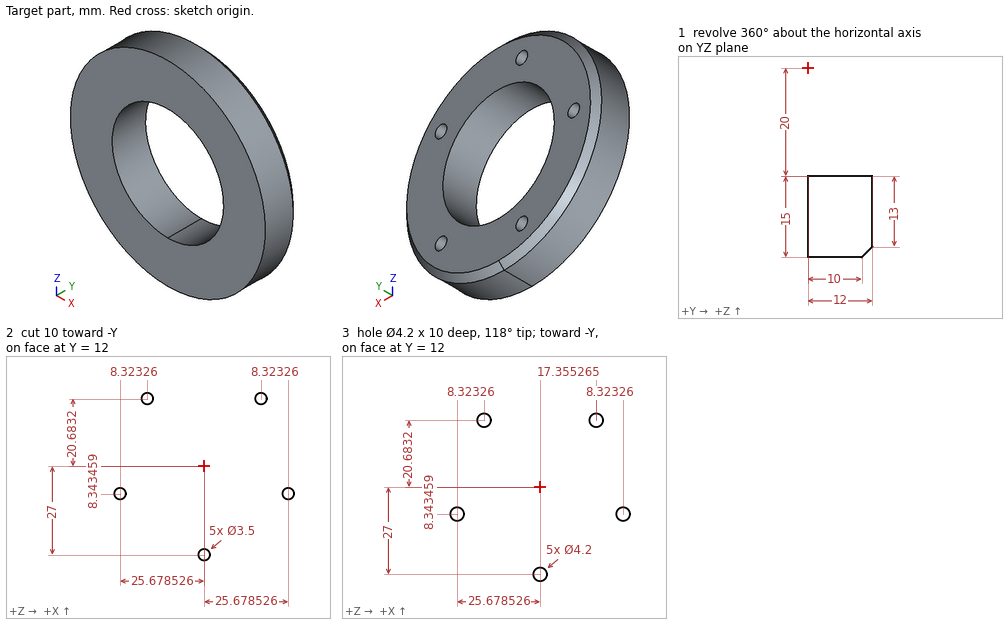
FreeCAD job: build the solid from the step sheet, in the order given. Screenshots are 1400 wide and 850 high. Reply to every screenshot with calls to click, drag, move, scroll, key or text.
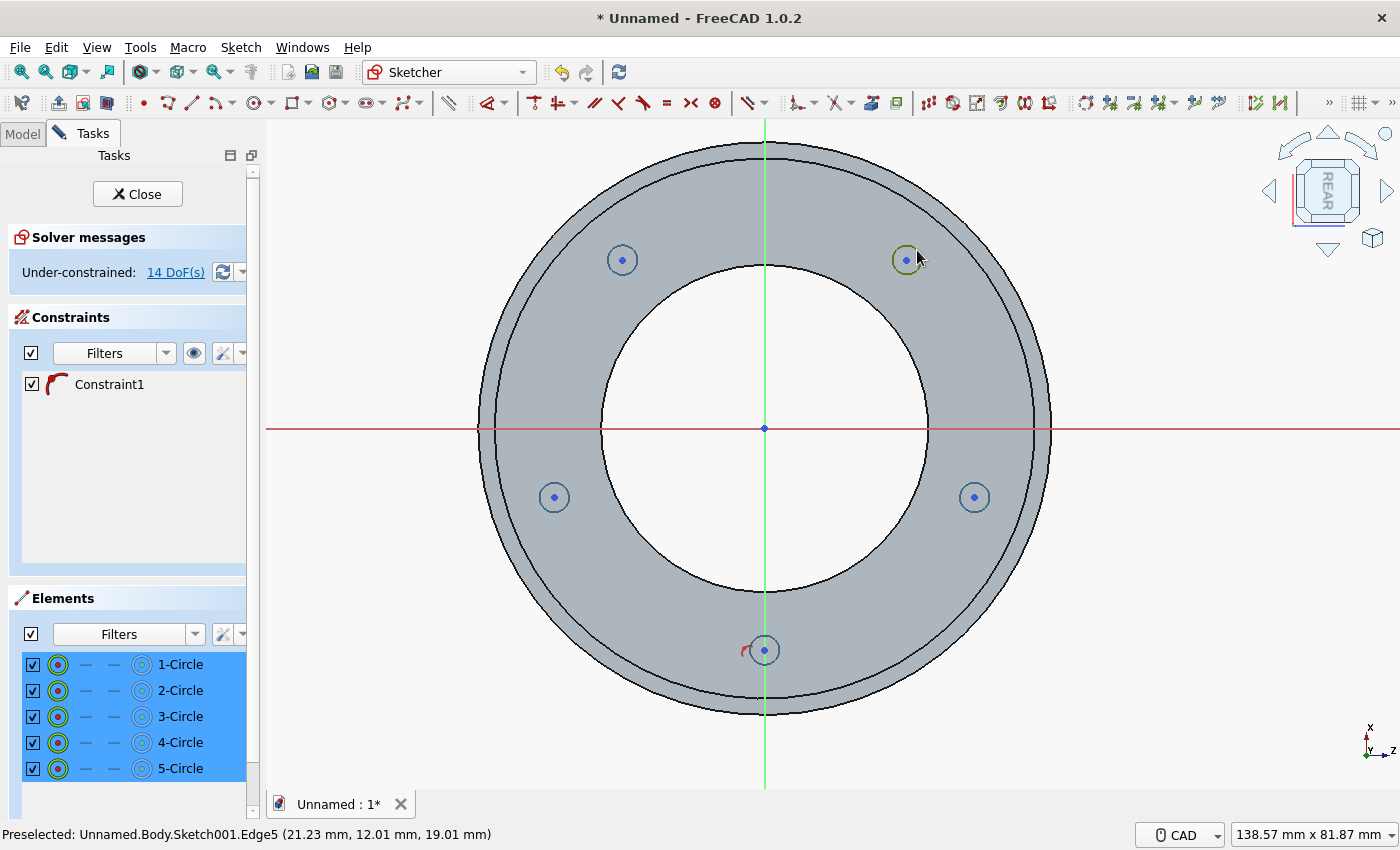
click(668, 104)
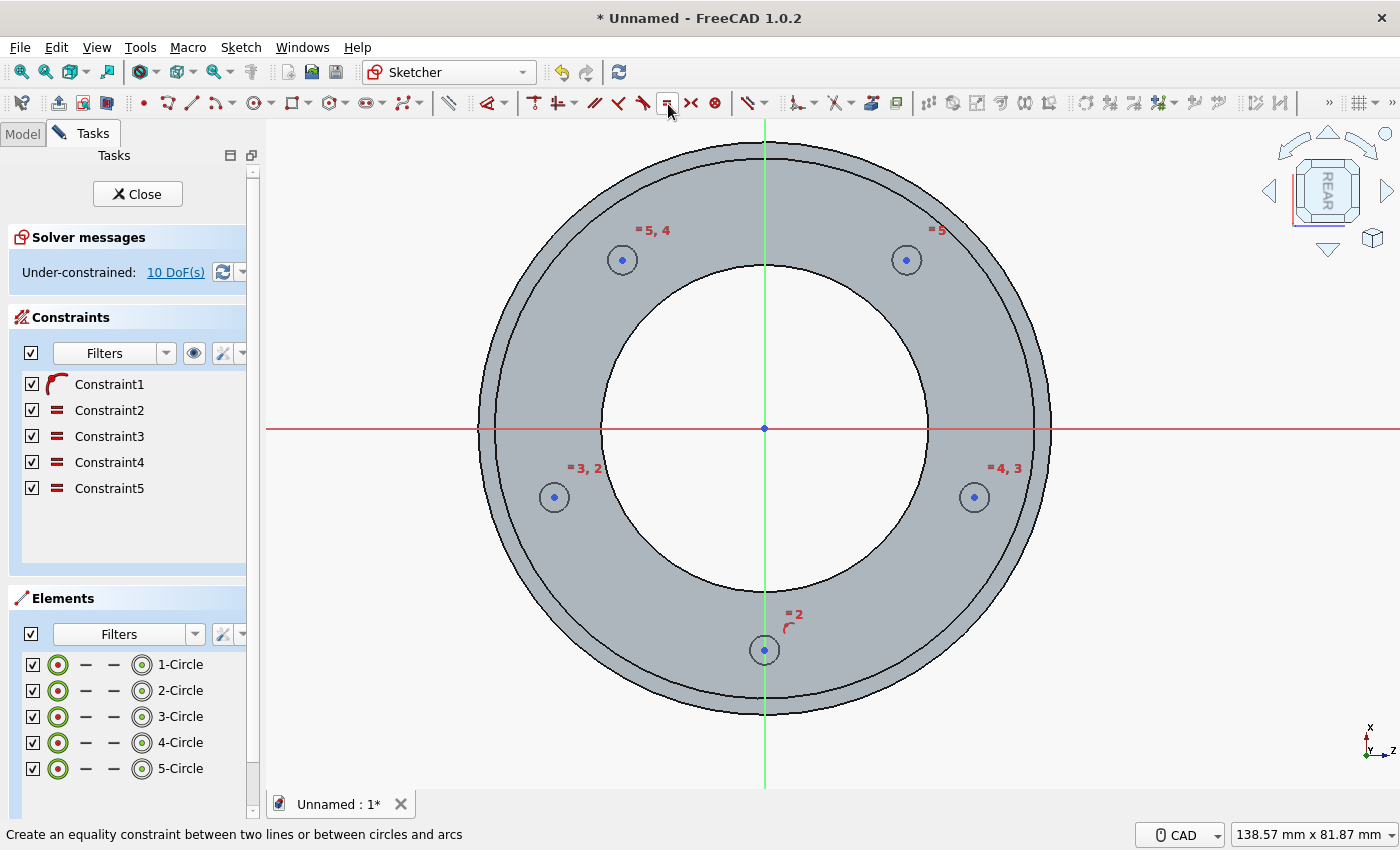
click(554, 498)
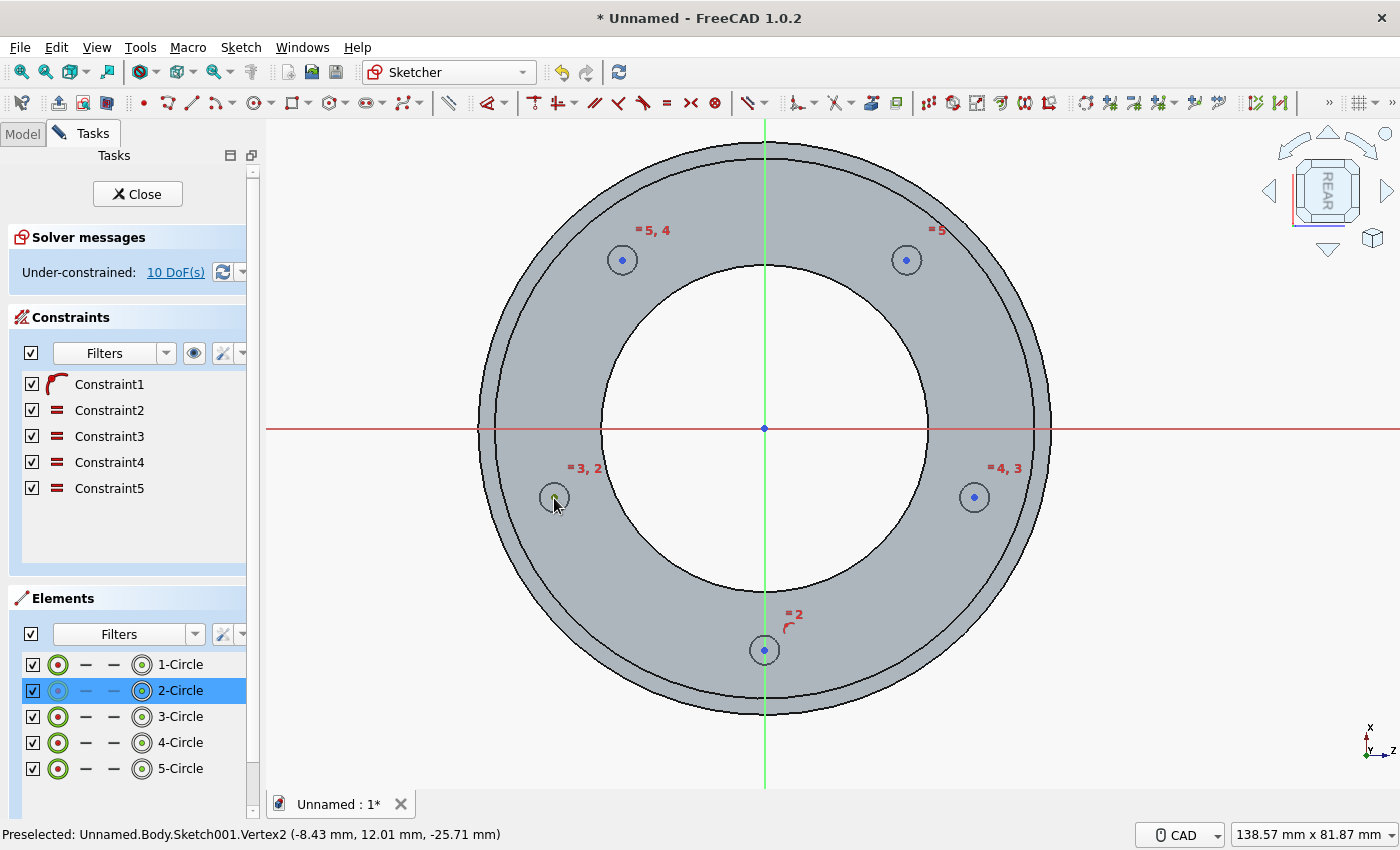
click(975, 498)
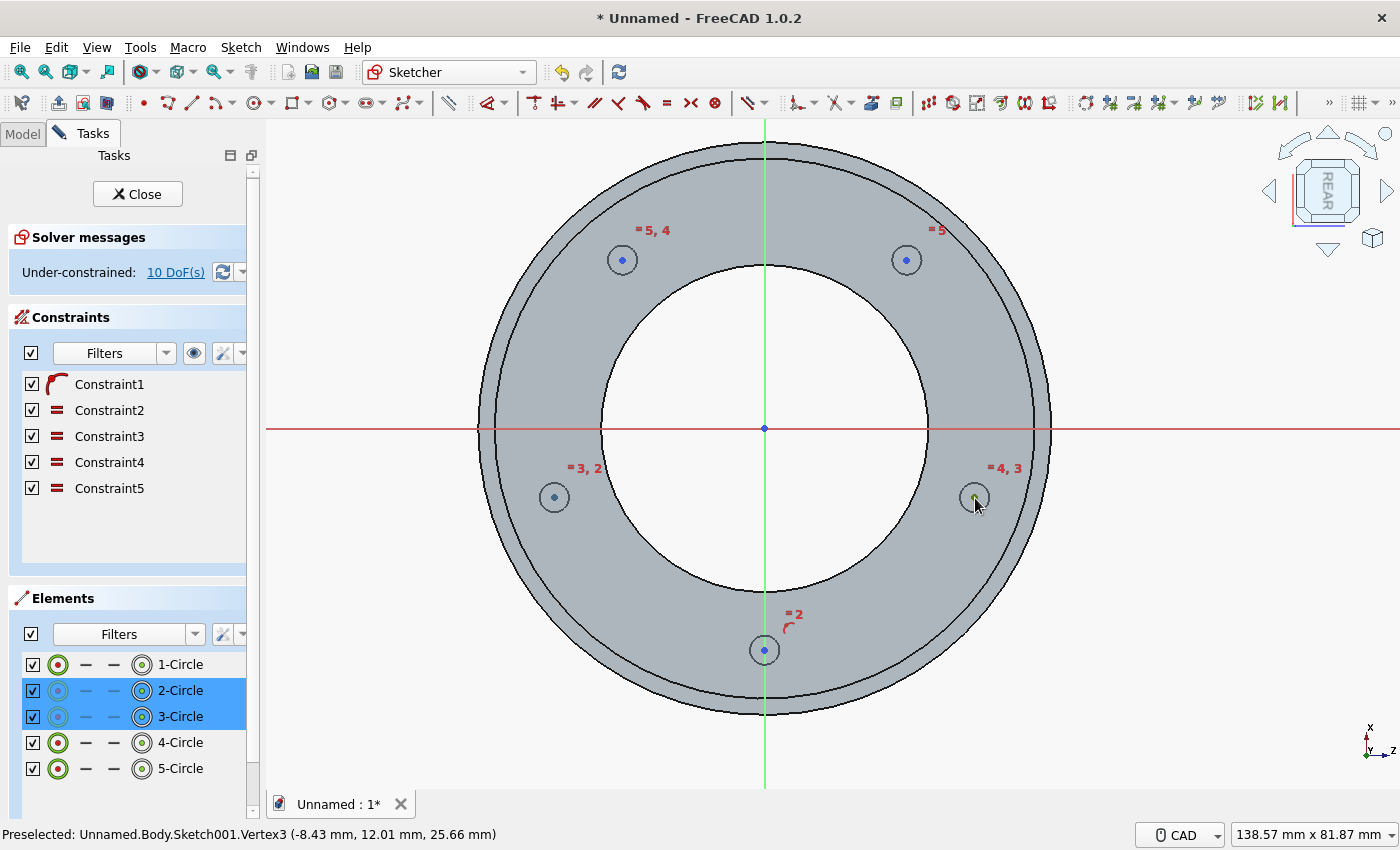
click(576, 104)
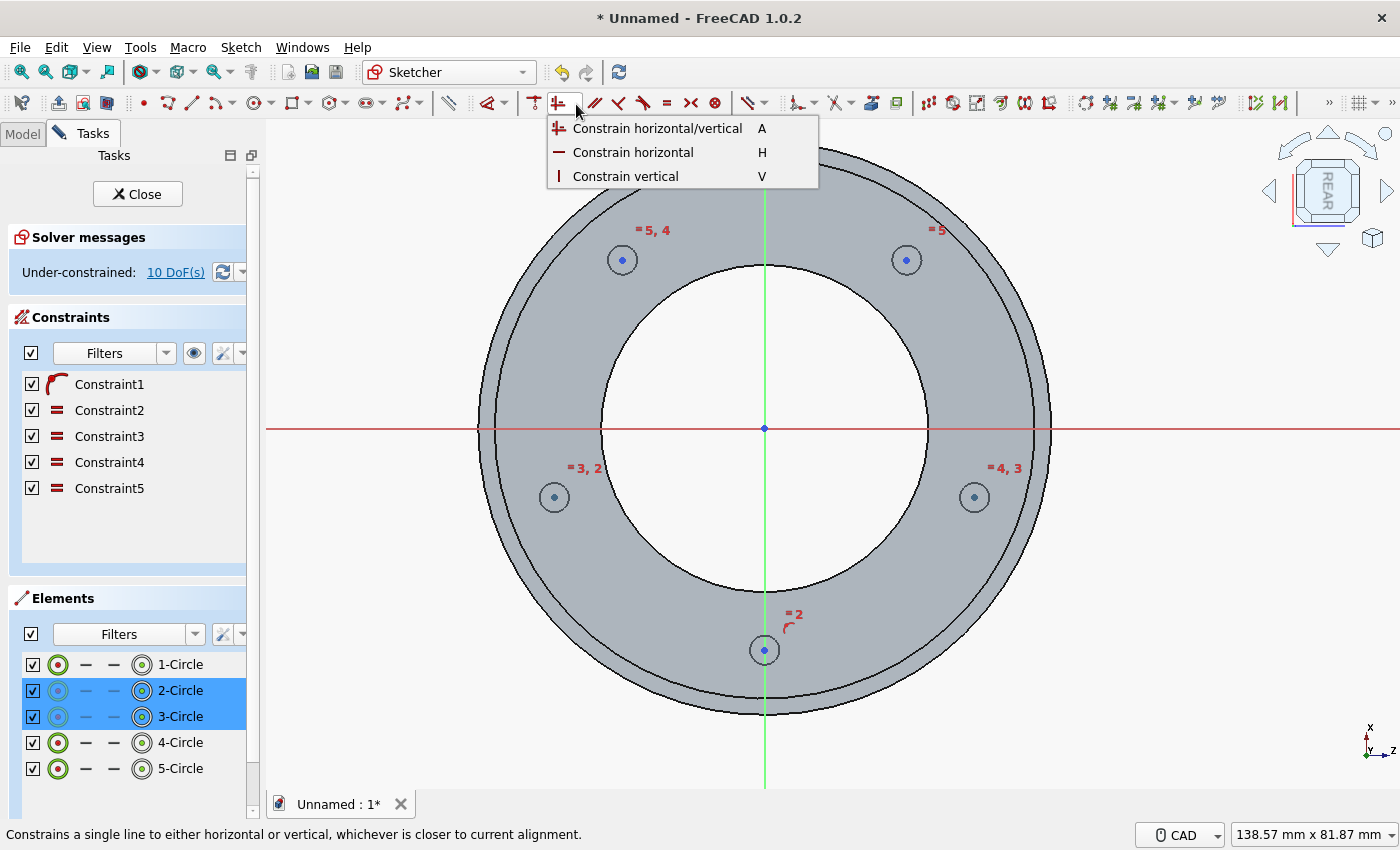
click(683, 152)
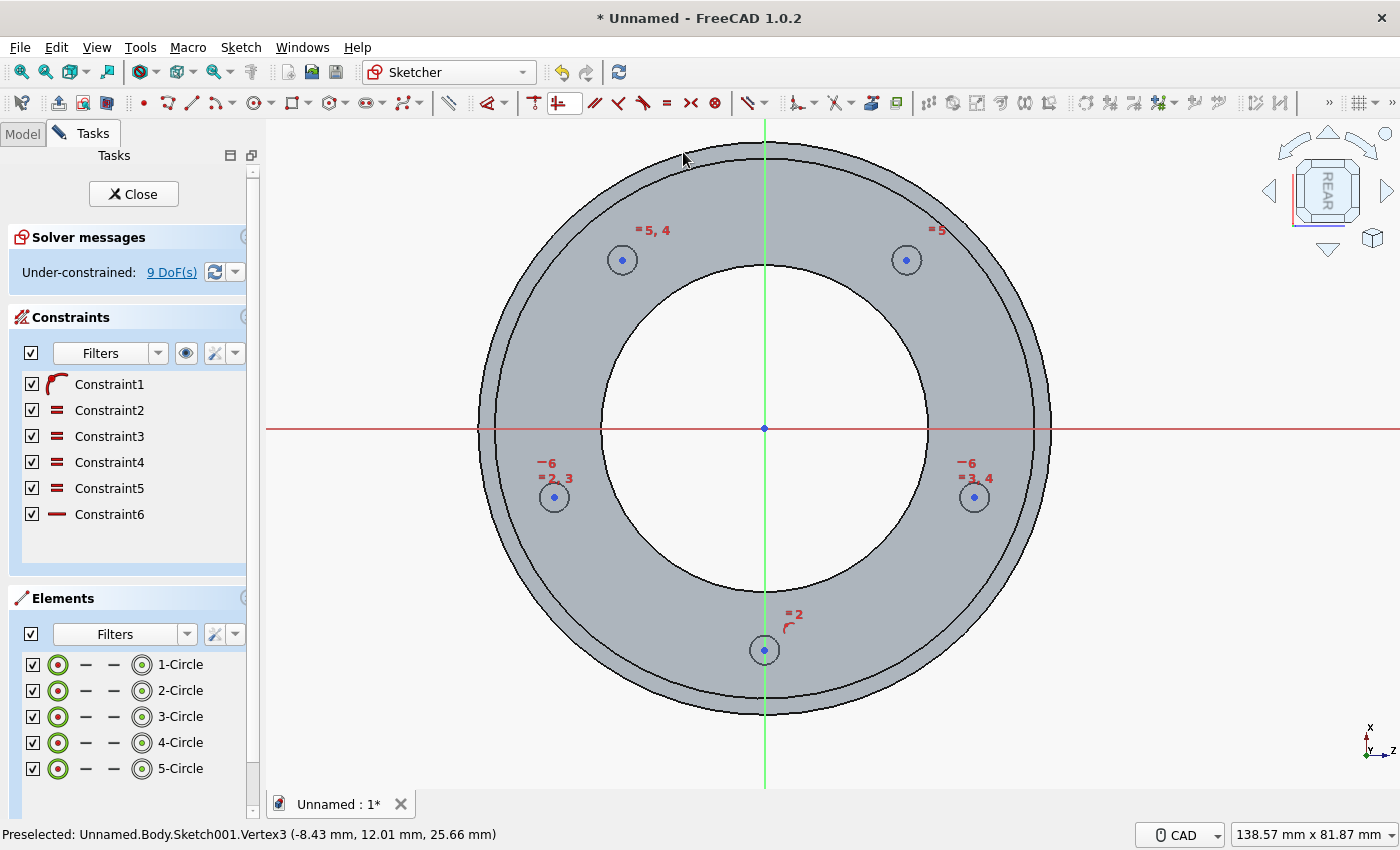
click(623, 260)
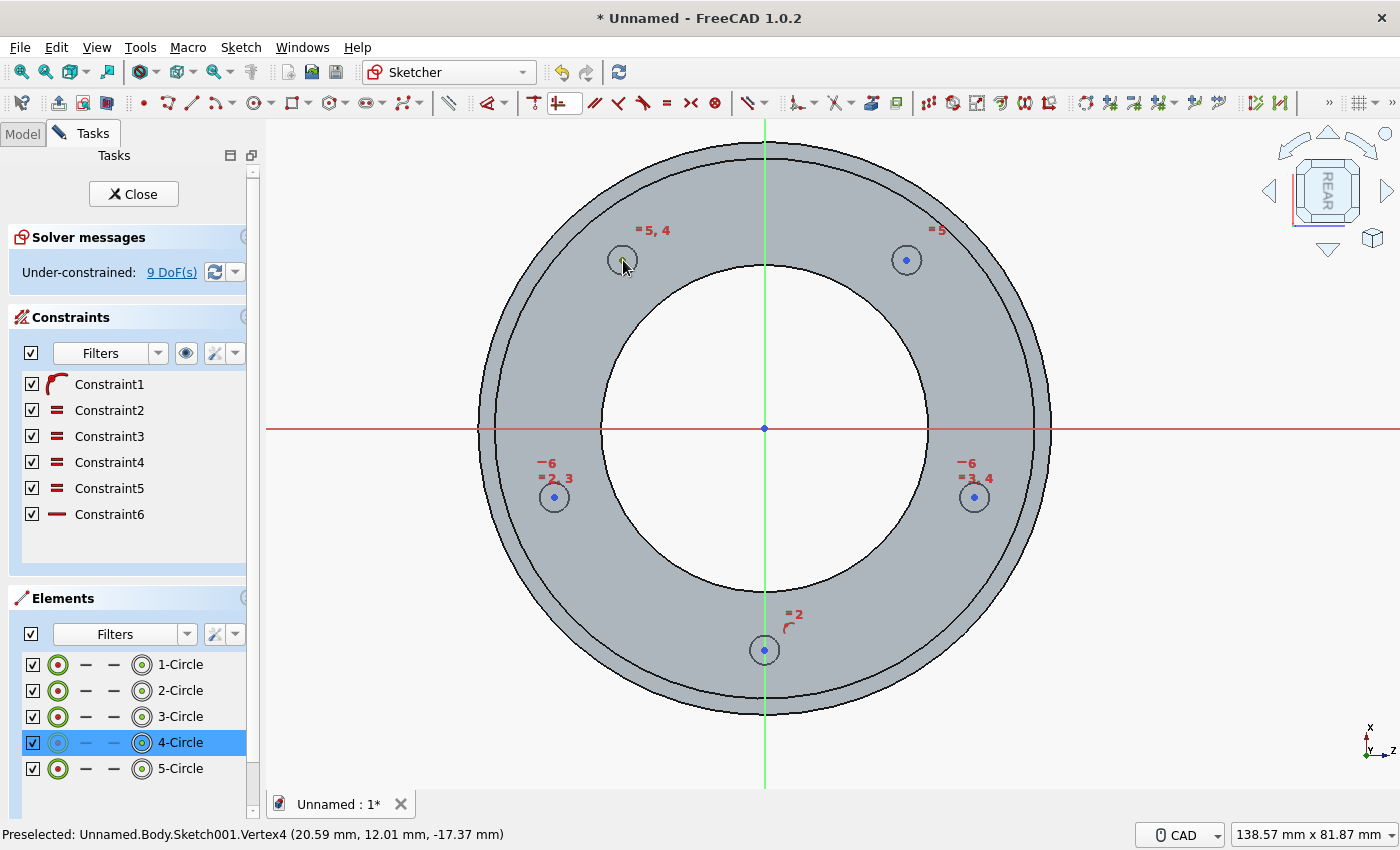
click(907, 260)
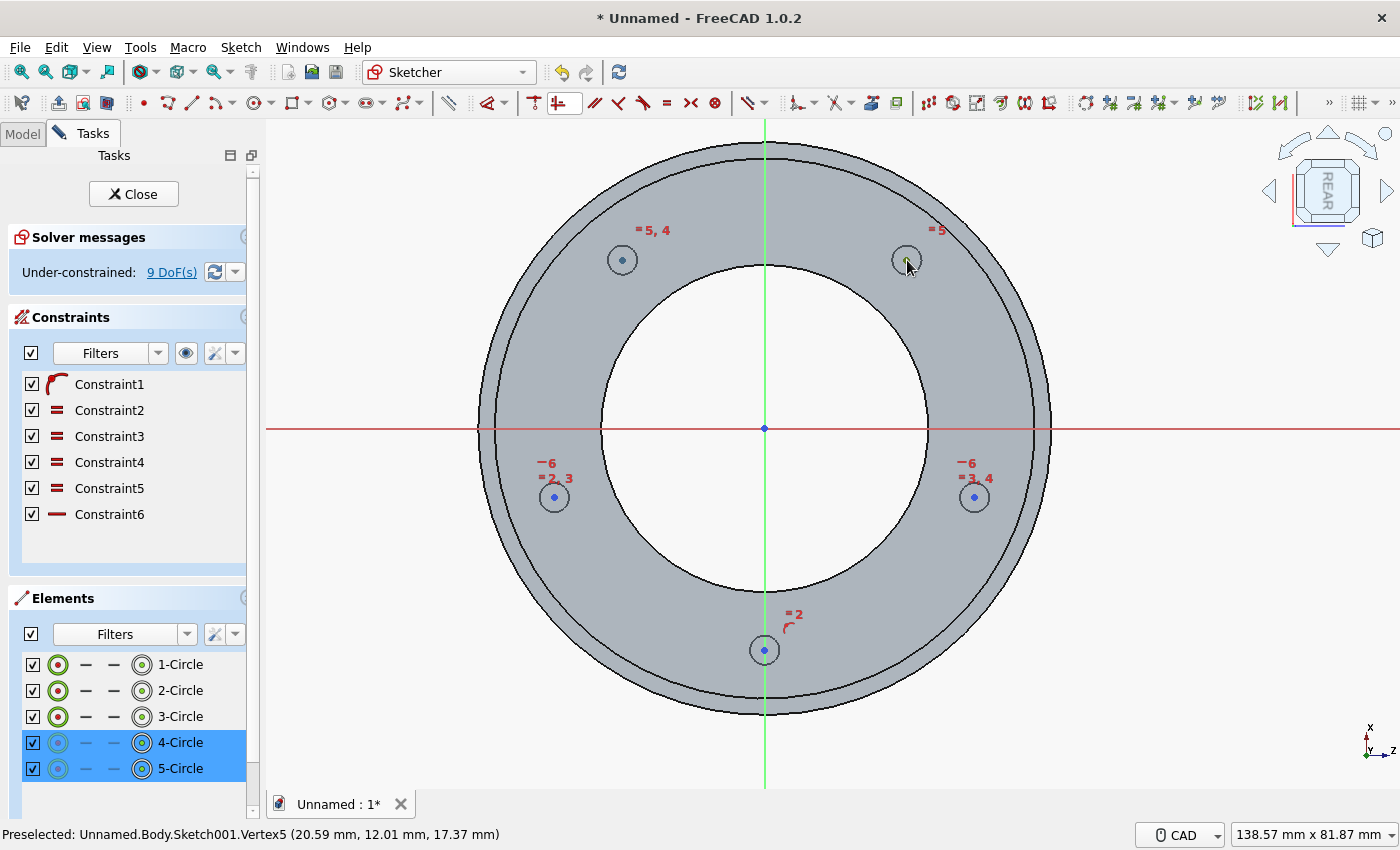
key(h)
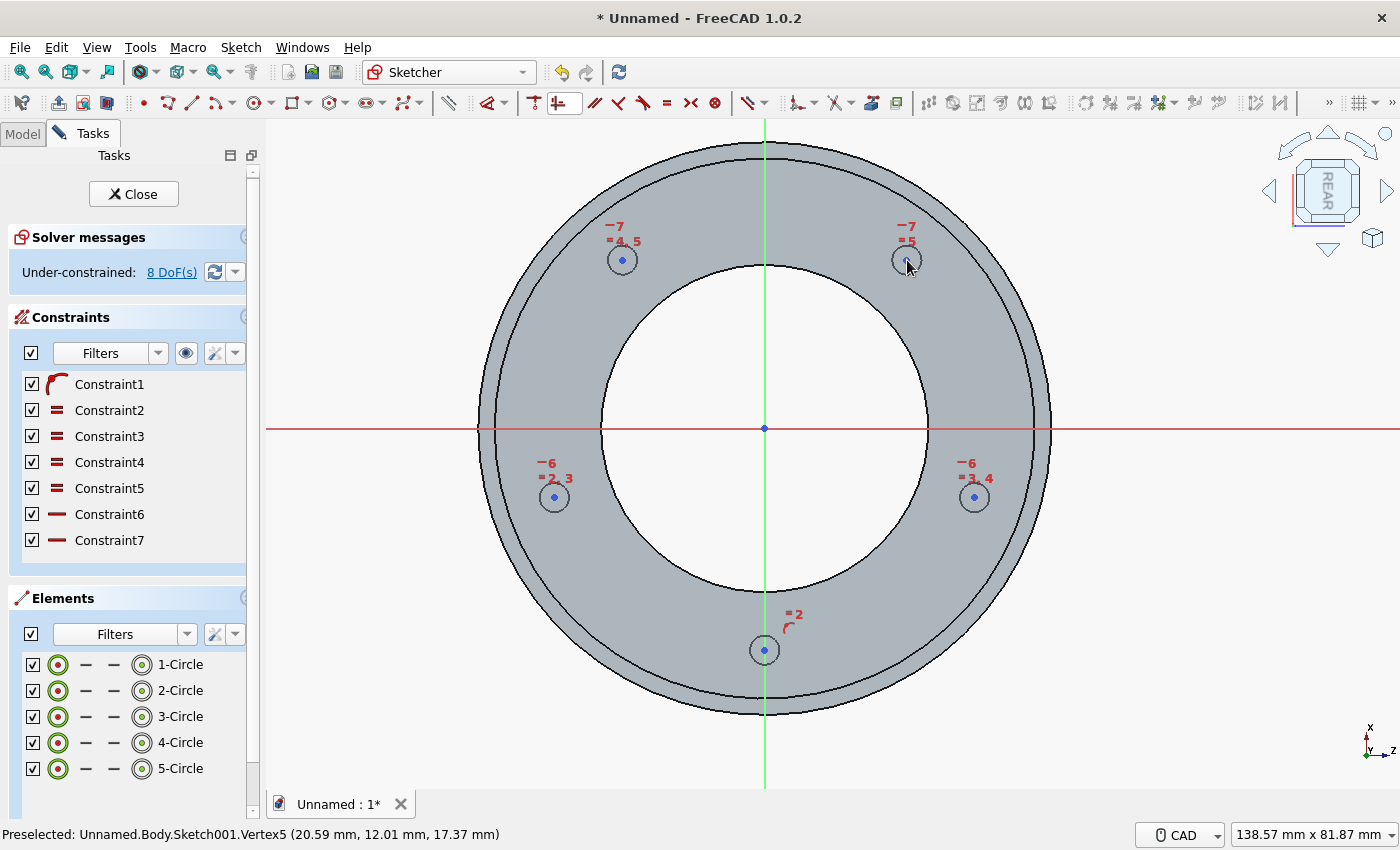
click(488, 104)